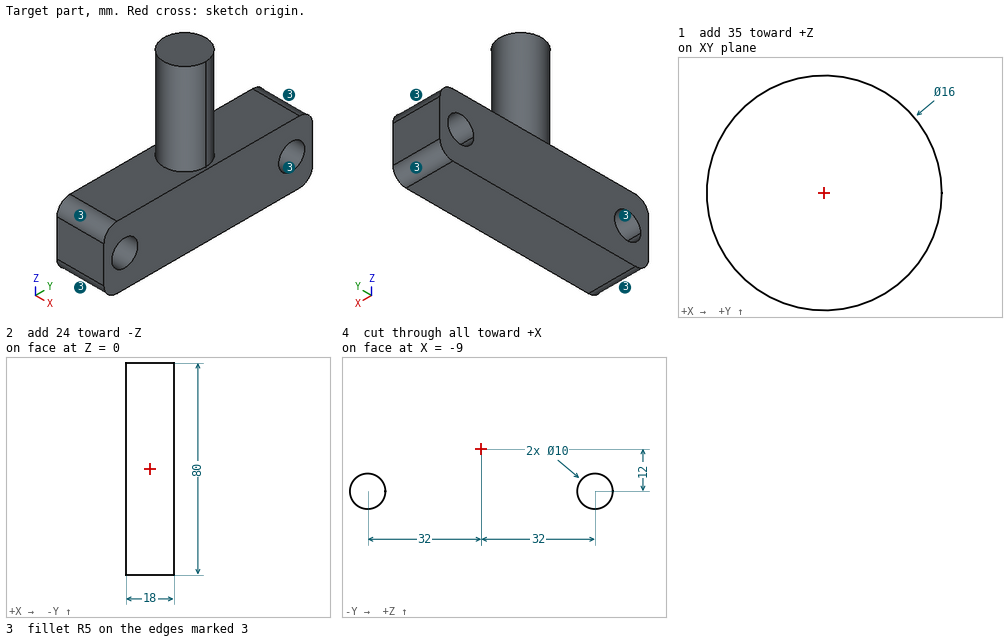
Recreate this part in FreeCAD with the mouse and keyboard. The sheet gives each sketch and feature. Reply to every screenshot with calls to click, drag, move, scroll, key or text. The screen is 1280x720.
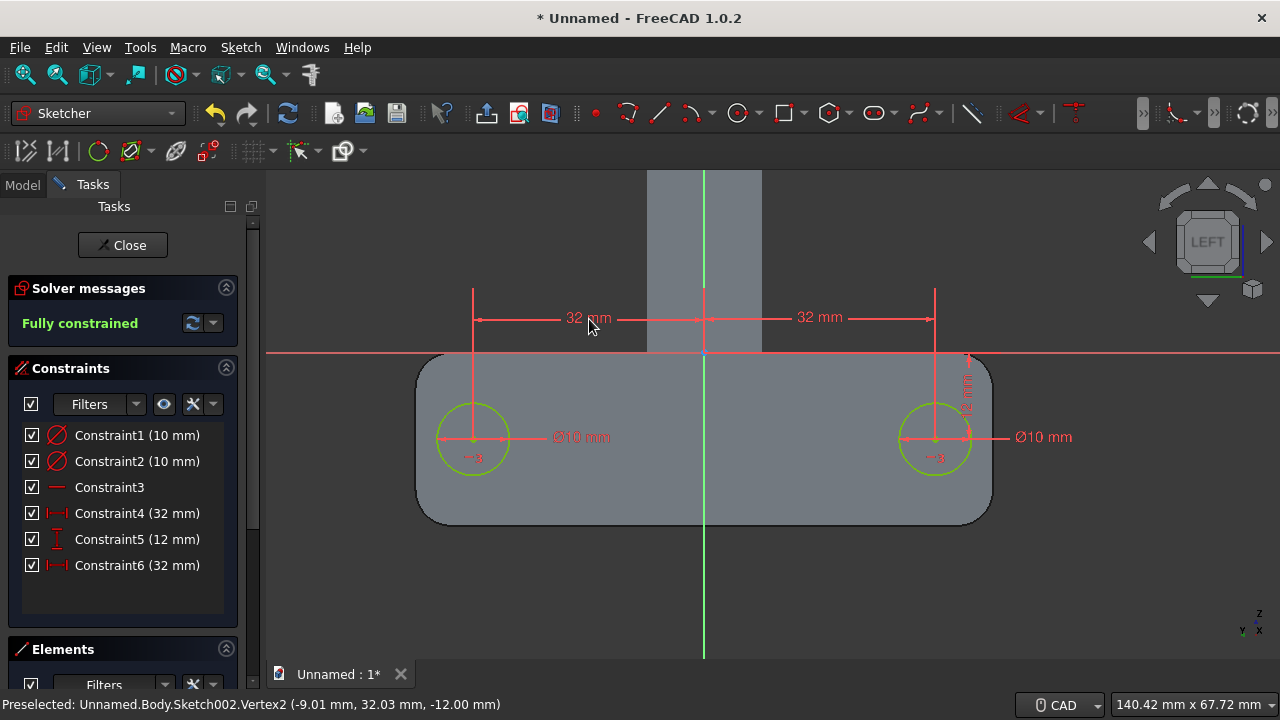
click(123, 245)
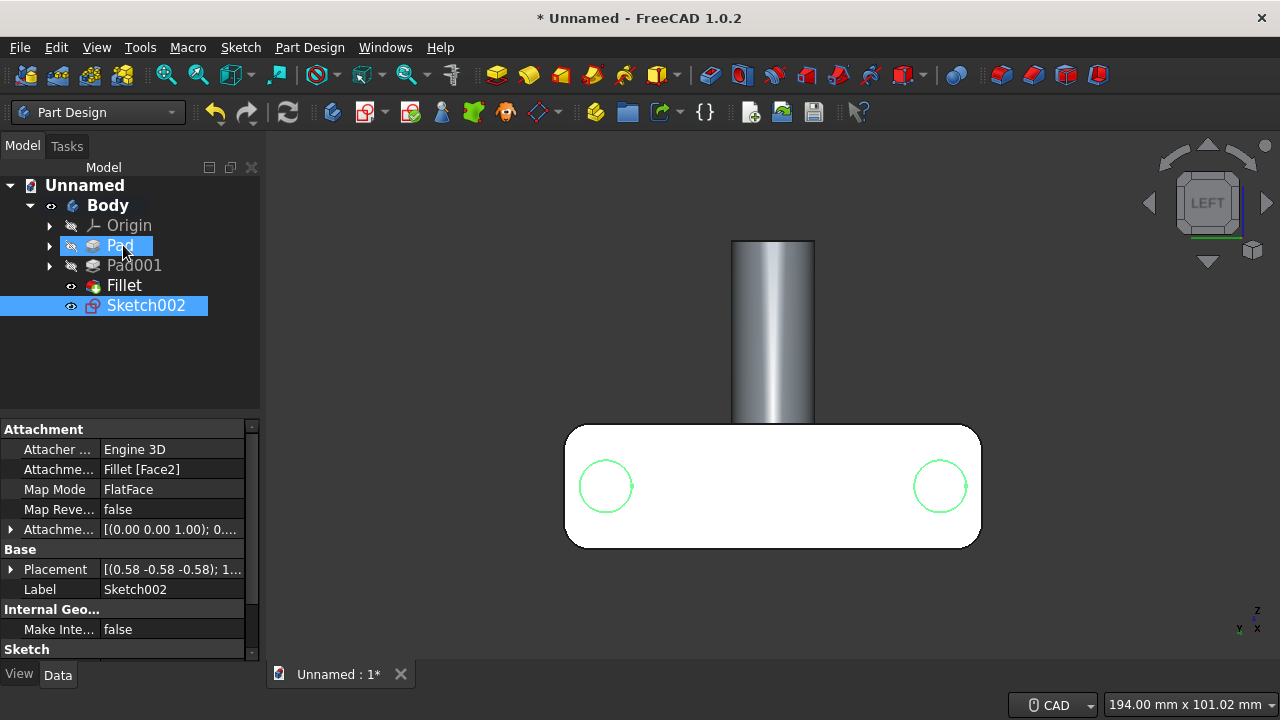
click(712, 76)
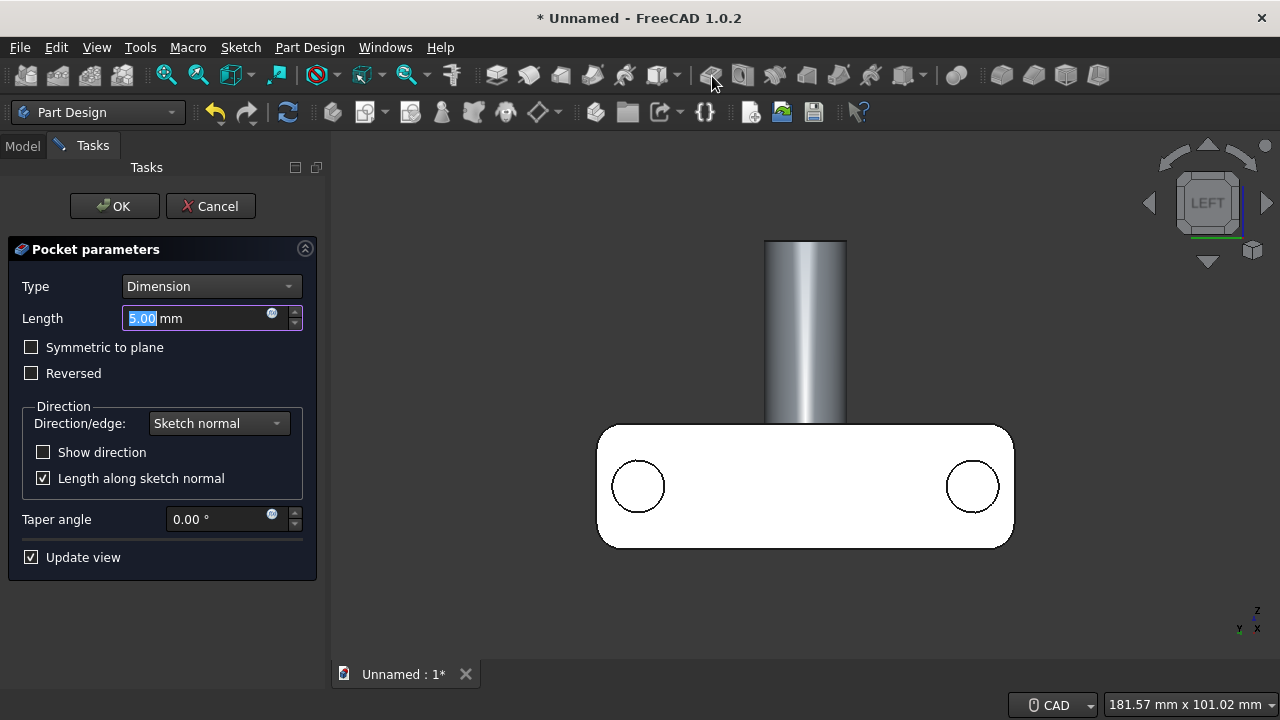
click(212, 286)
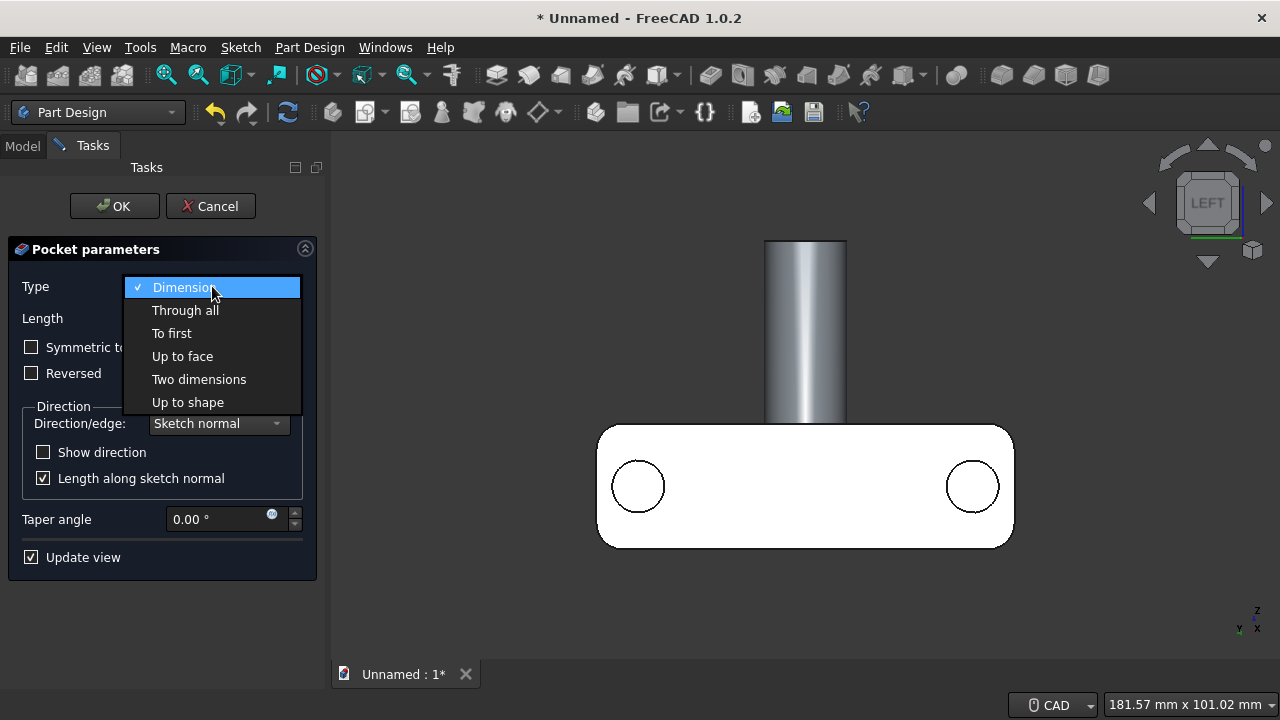
click(212, 310)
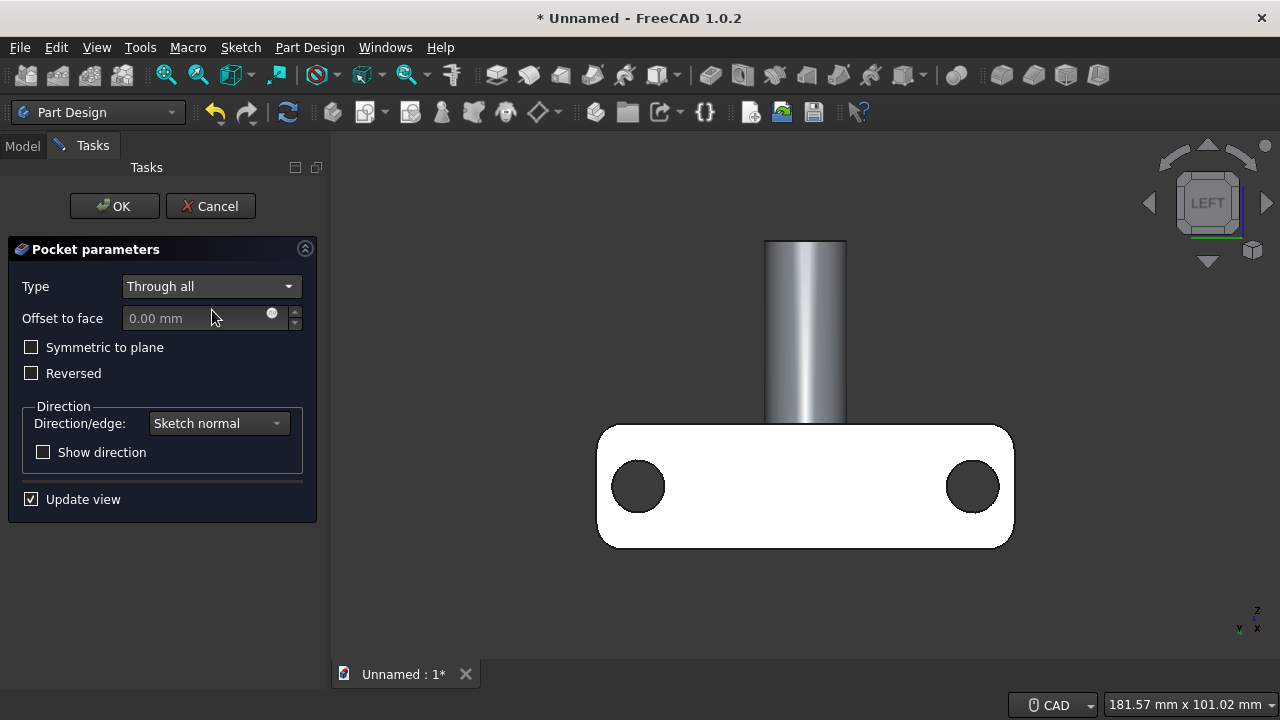
click(115, 206)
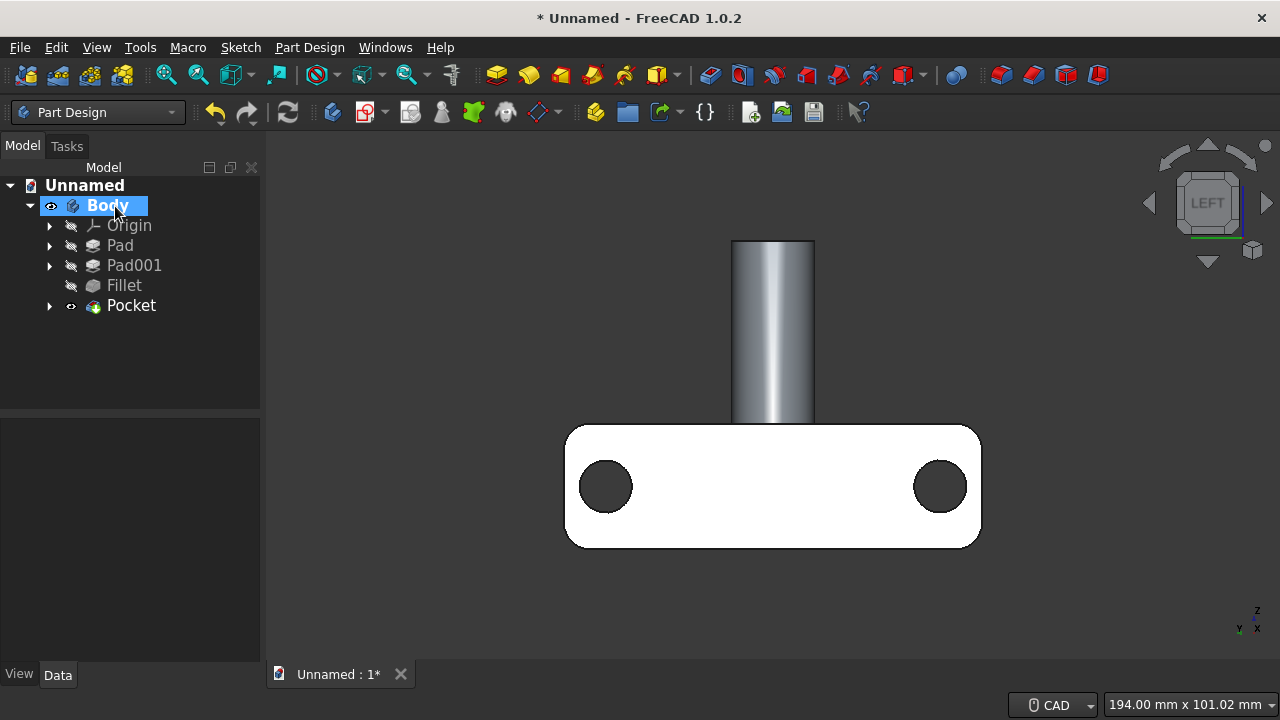
key(0)